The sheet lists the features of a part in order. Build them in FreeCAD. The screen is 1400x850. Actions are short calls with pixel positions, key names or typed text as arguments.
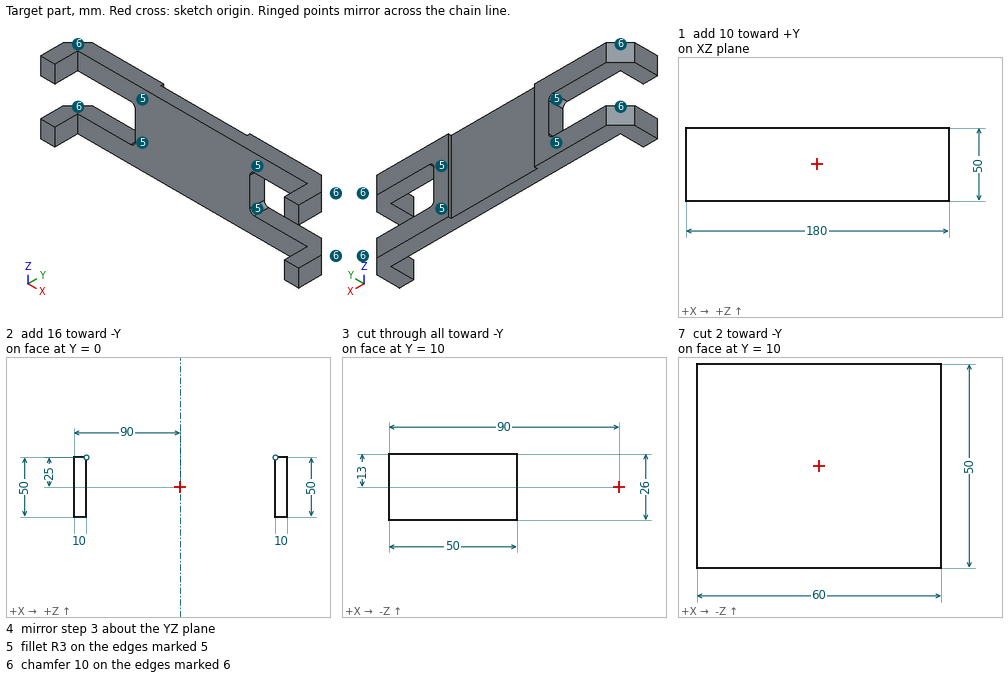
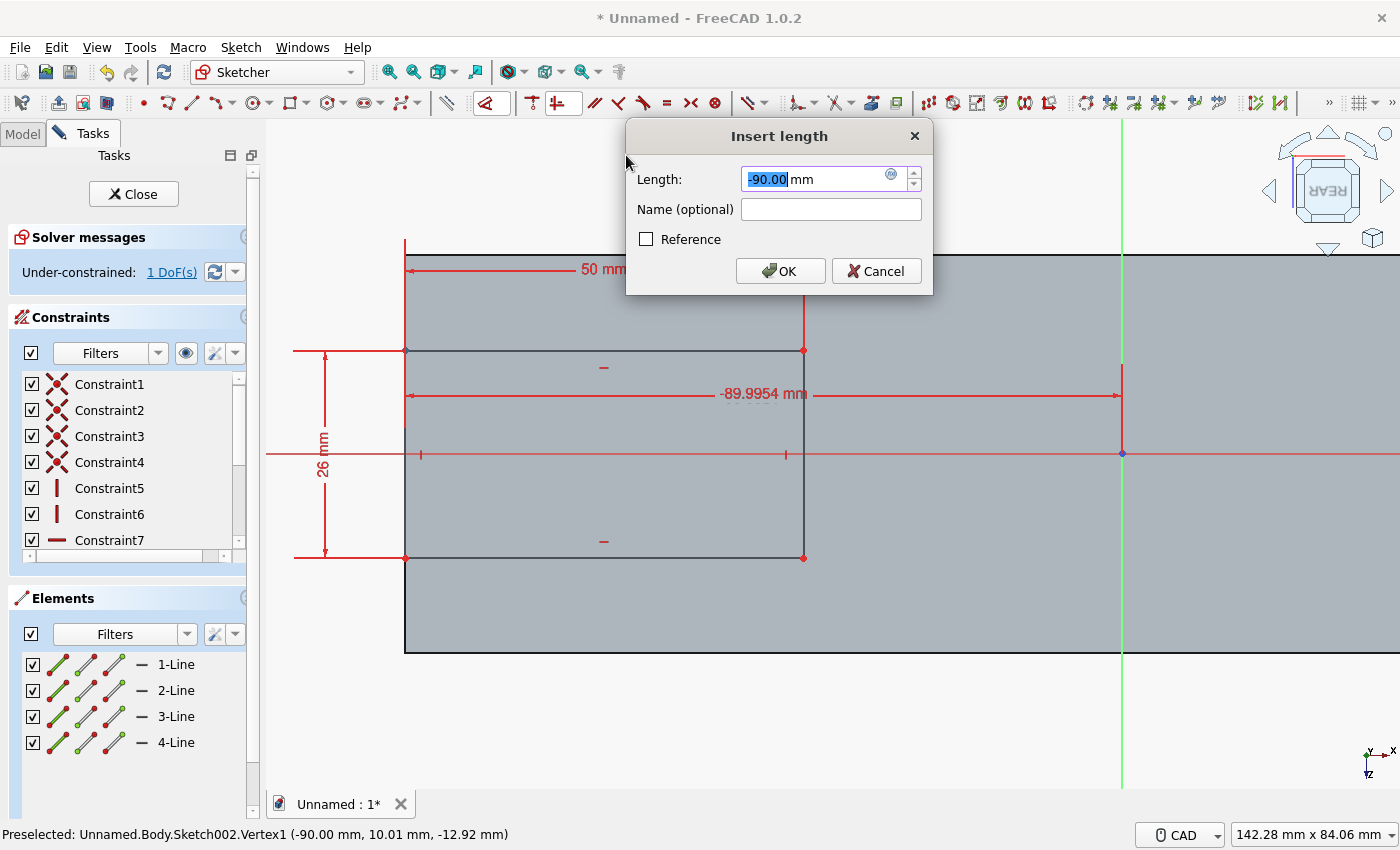
text(-90)
key(Return)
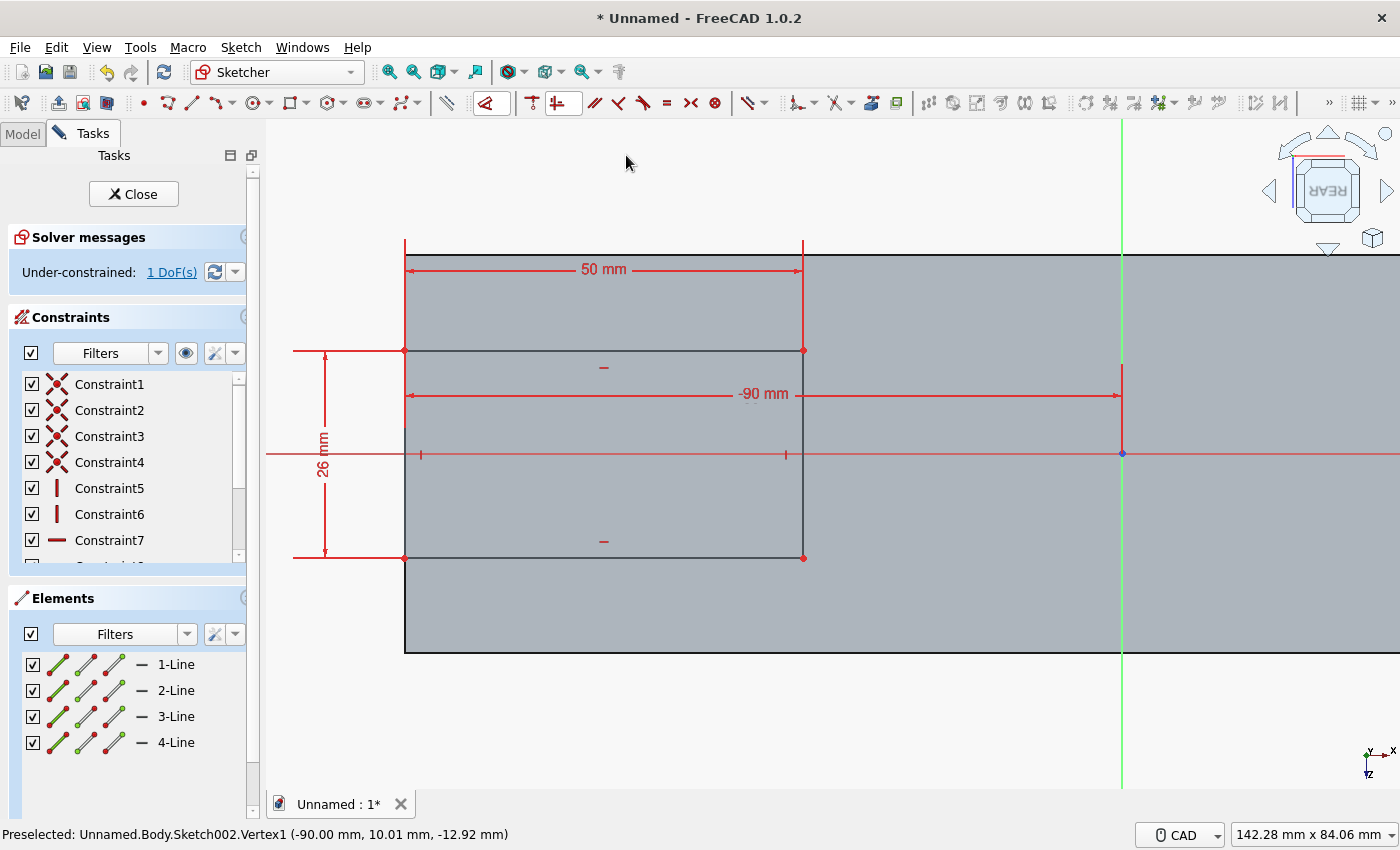
click(405, 351)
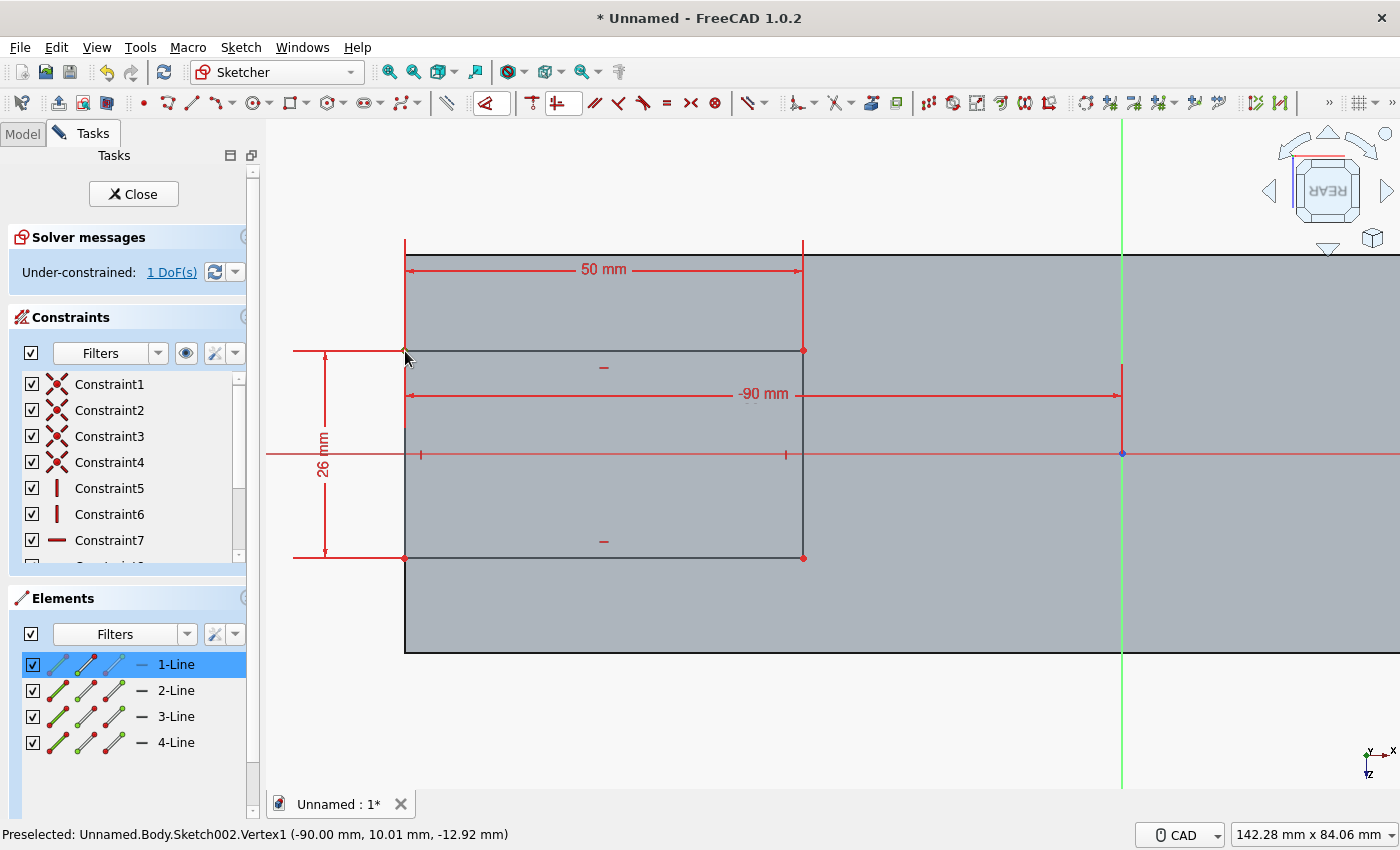
key(i)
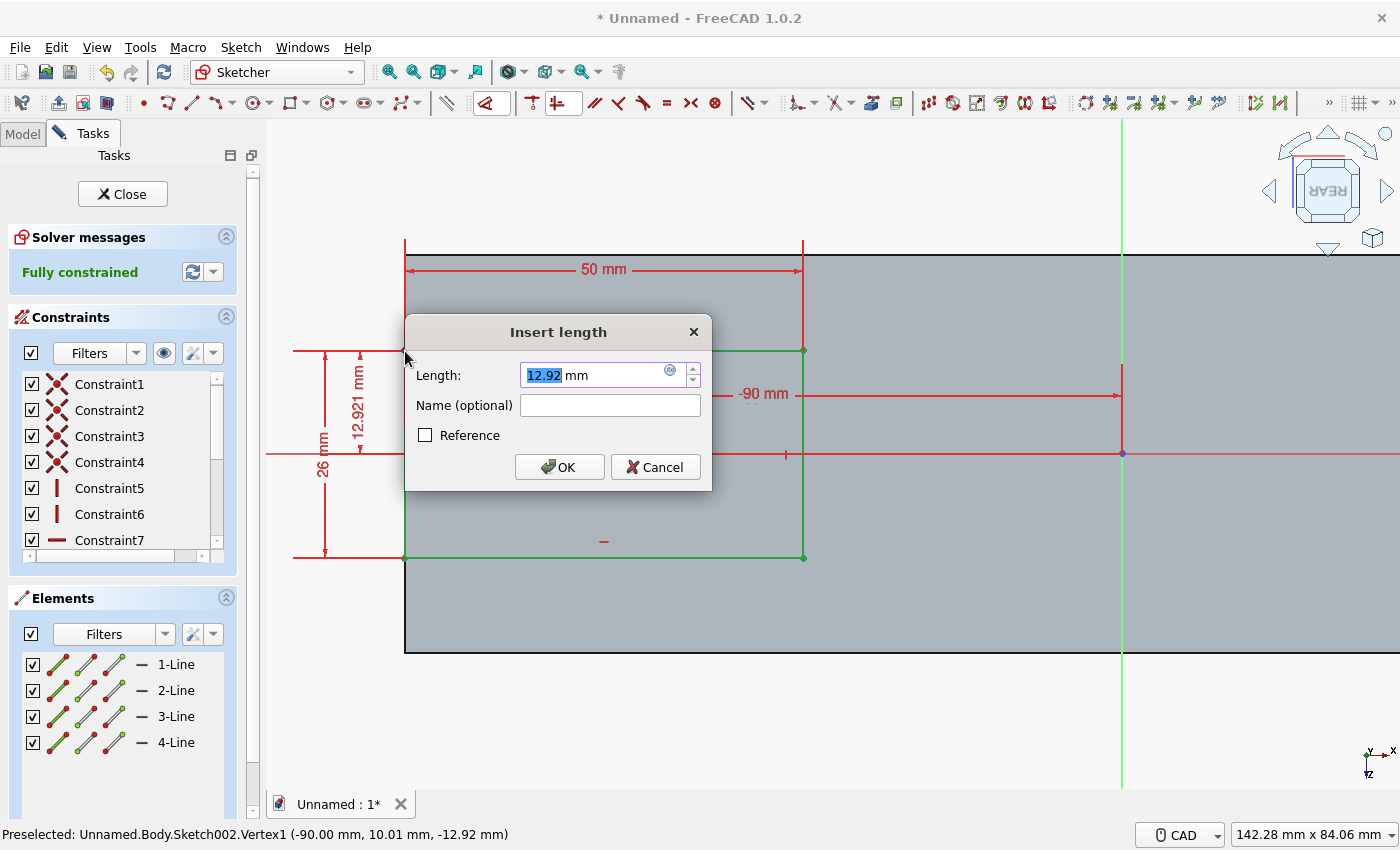
text(13)
key(Return)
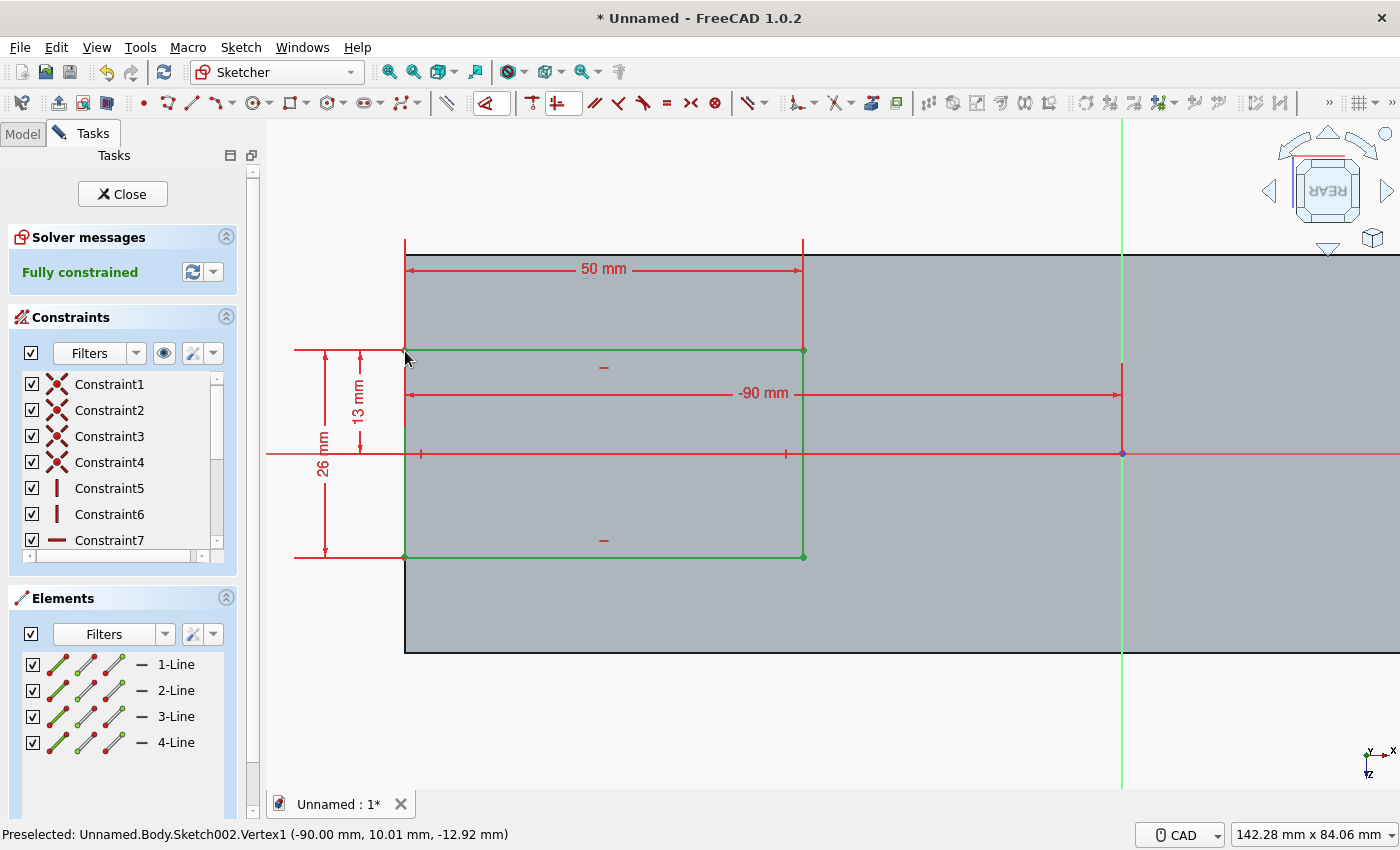
click(123, 194)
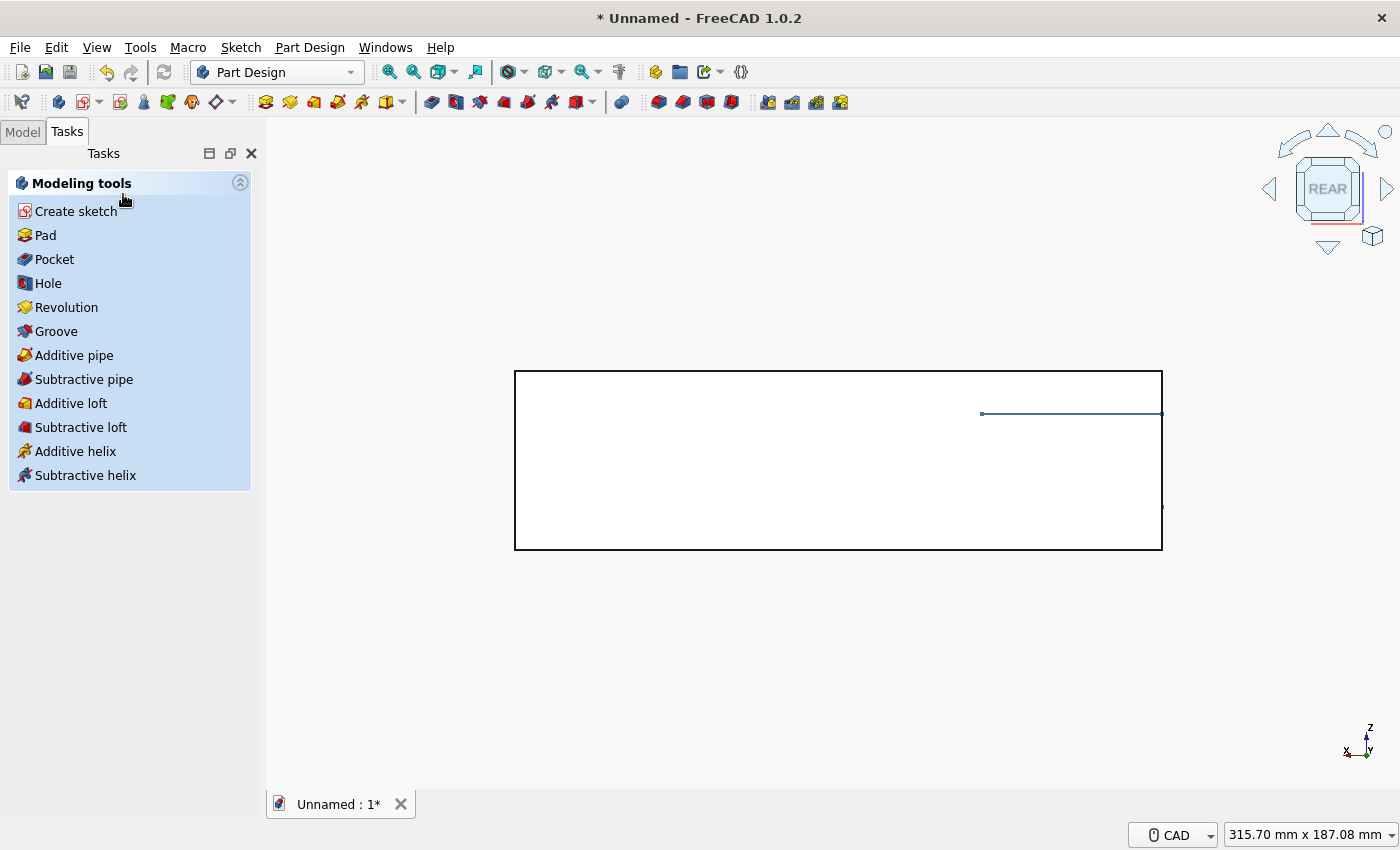
click(432, 102)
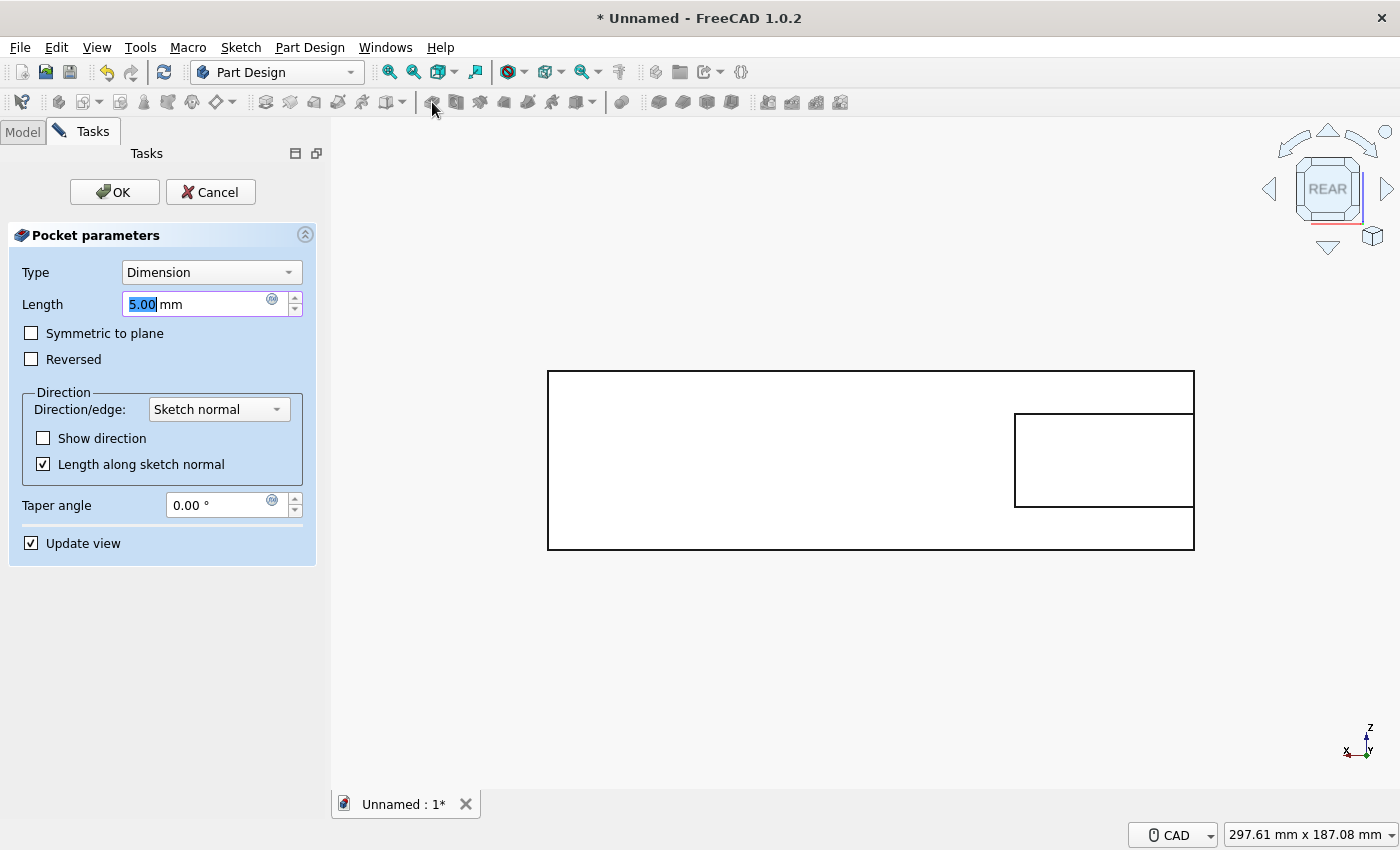
click(212, 272)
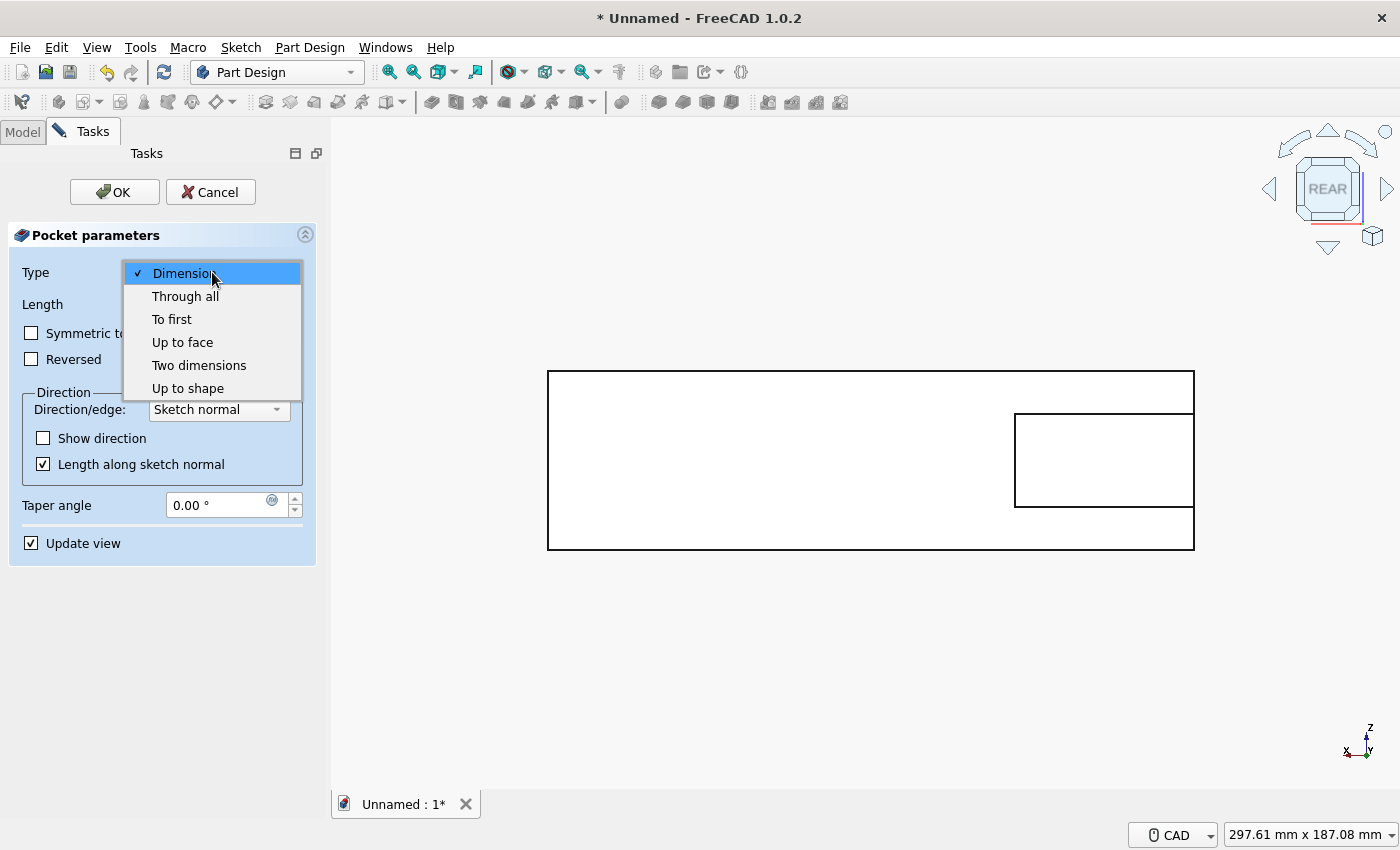
click(212, 296)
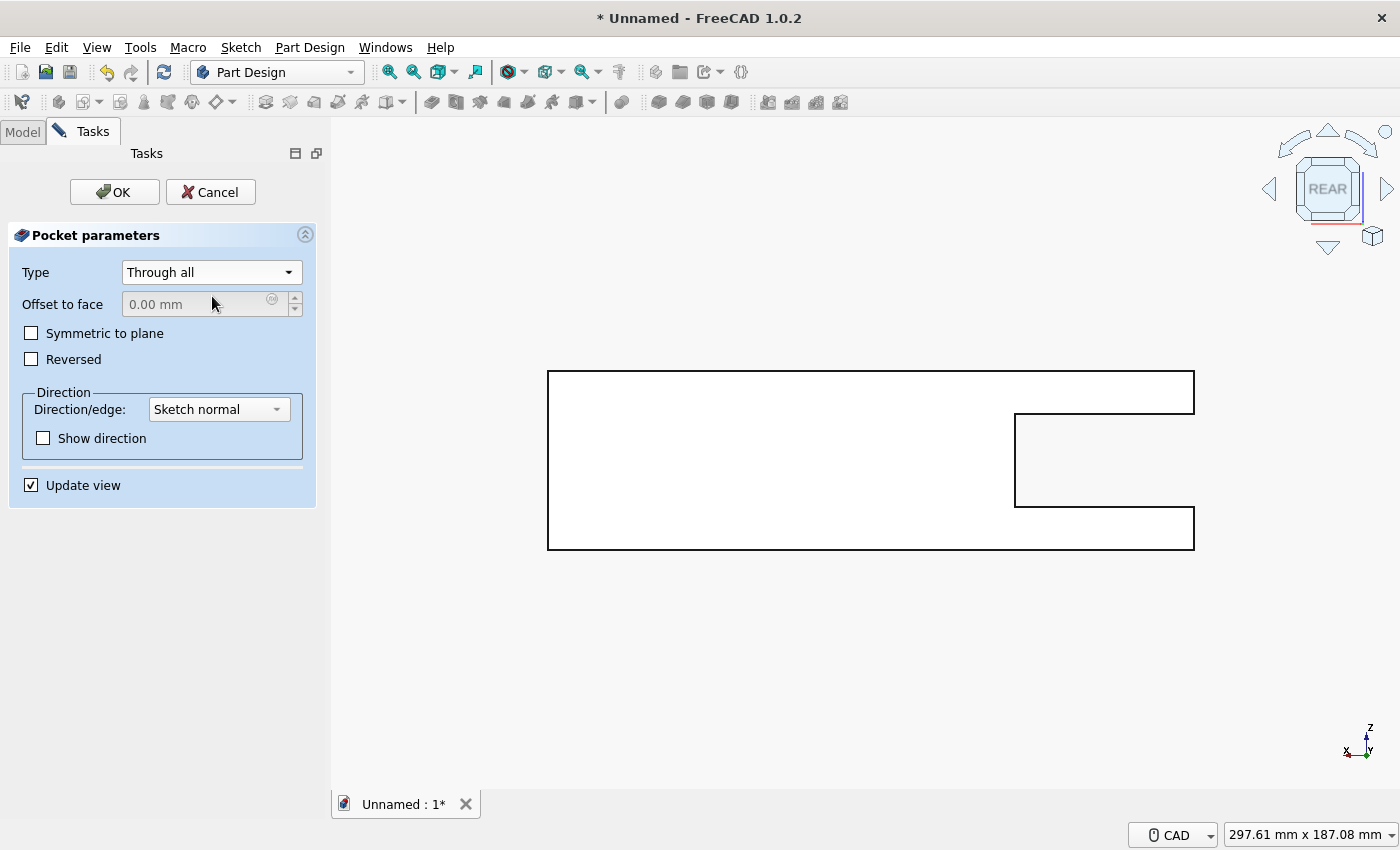
click(115, 192)